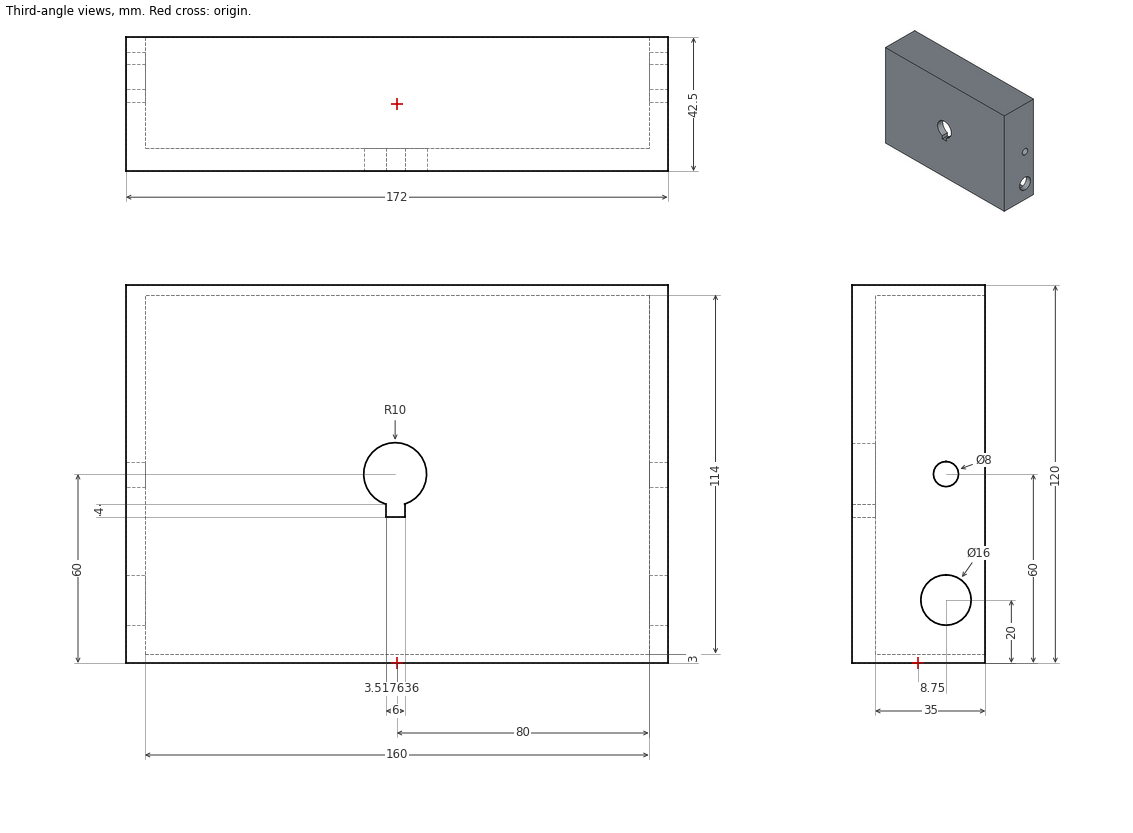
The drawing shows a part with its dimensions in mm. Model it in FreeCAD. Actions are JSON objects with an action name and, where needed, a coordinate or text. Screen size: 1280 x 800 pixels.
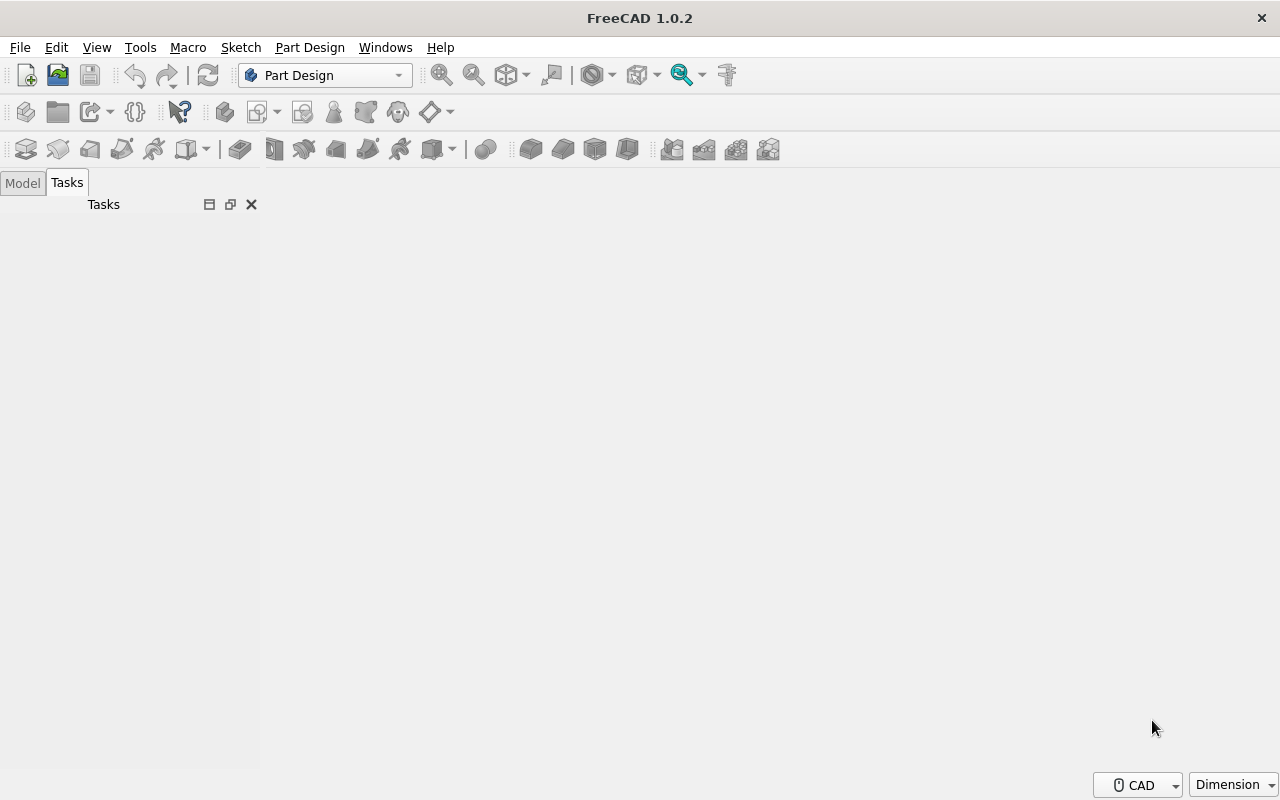
{"action": "left_click", "coordinate": [26, 76]}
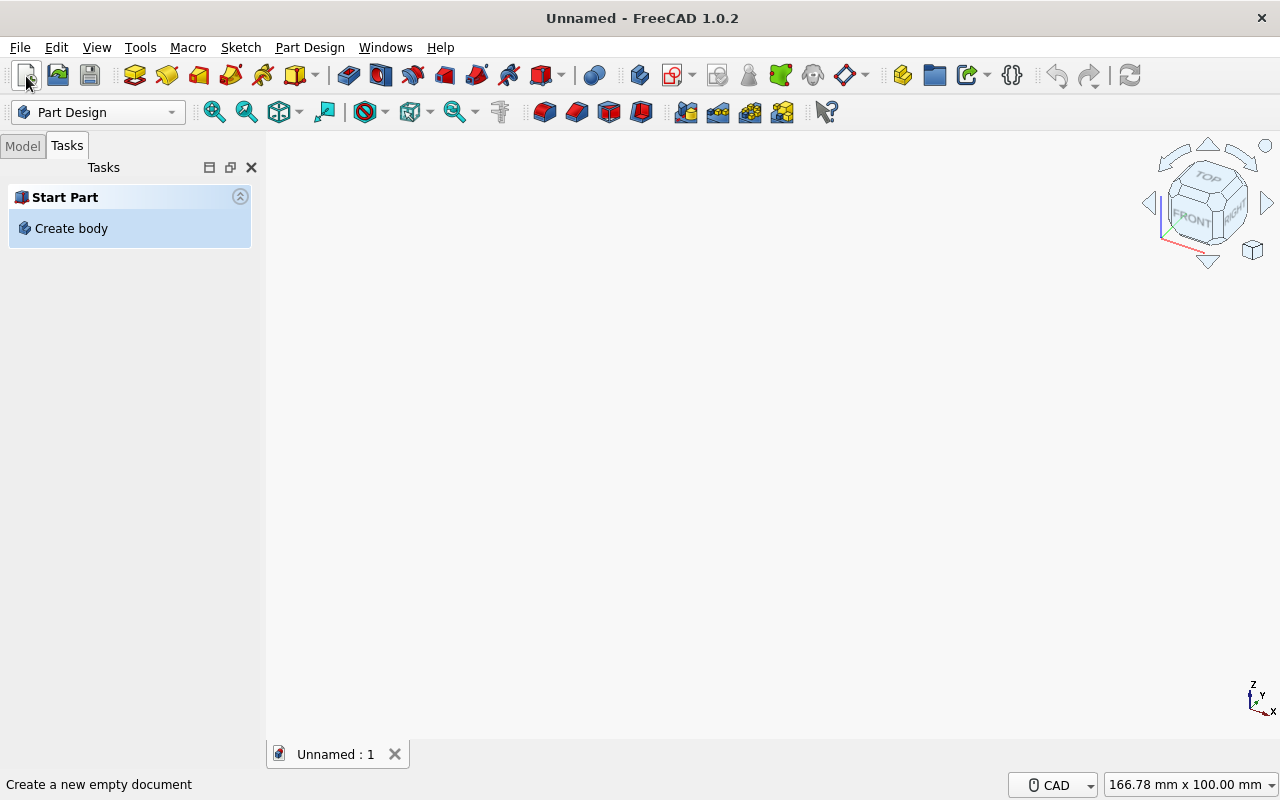
{"action": "left_click", "coordinate": [672, 76]}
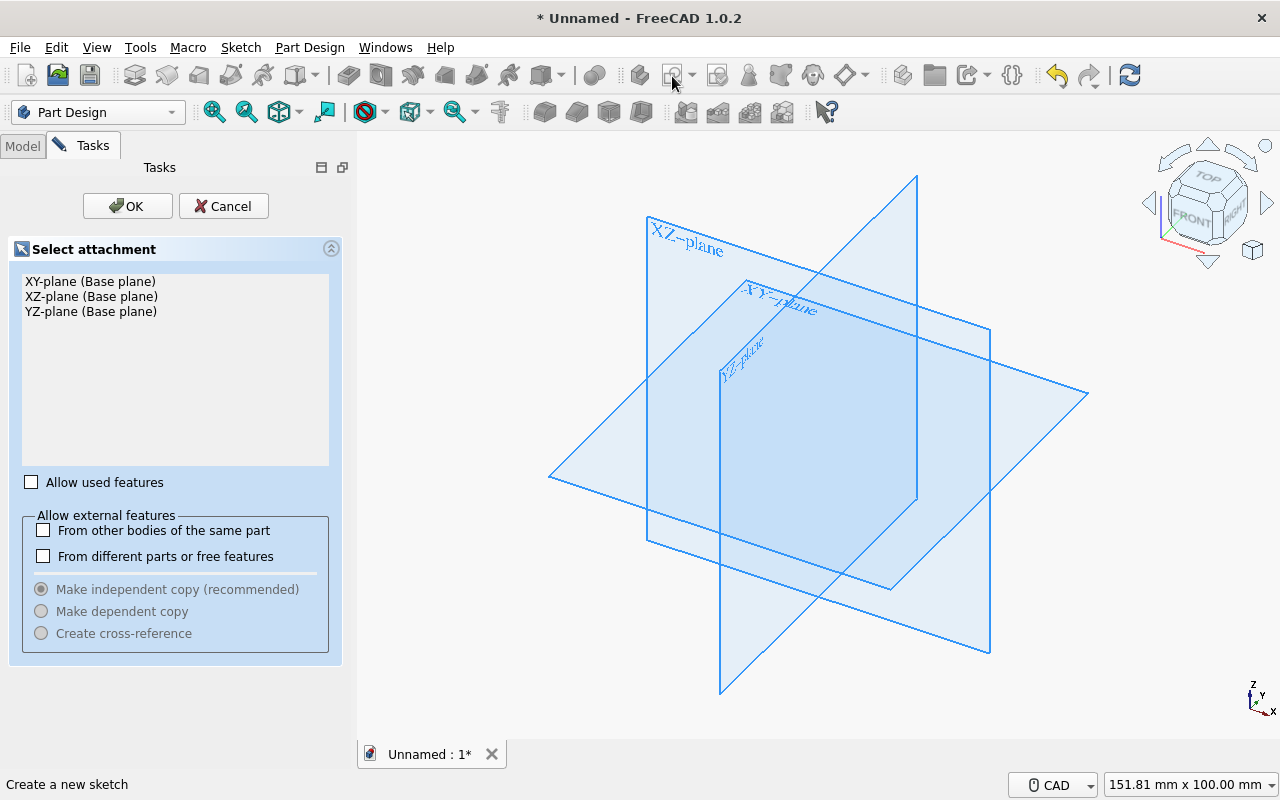
{"action": "left_click", "coordinate": [82, 282]}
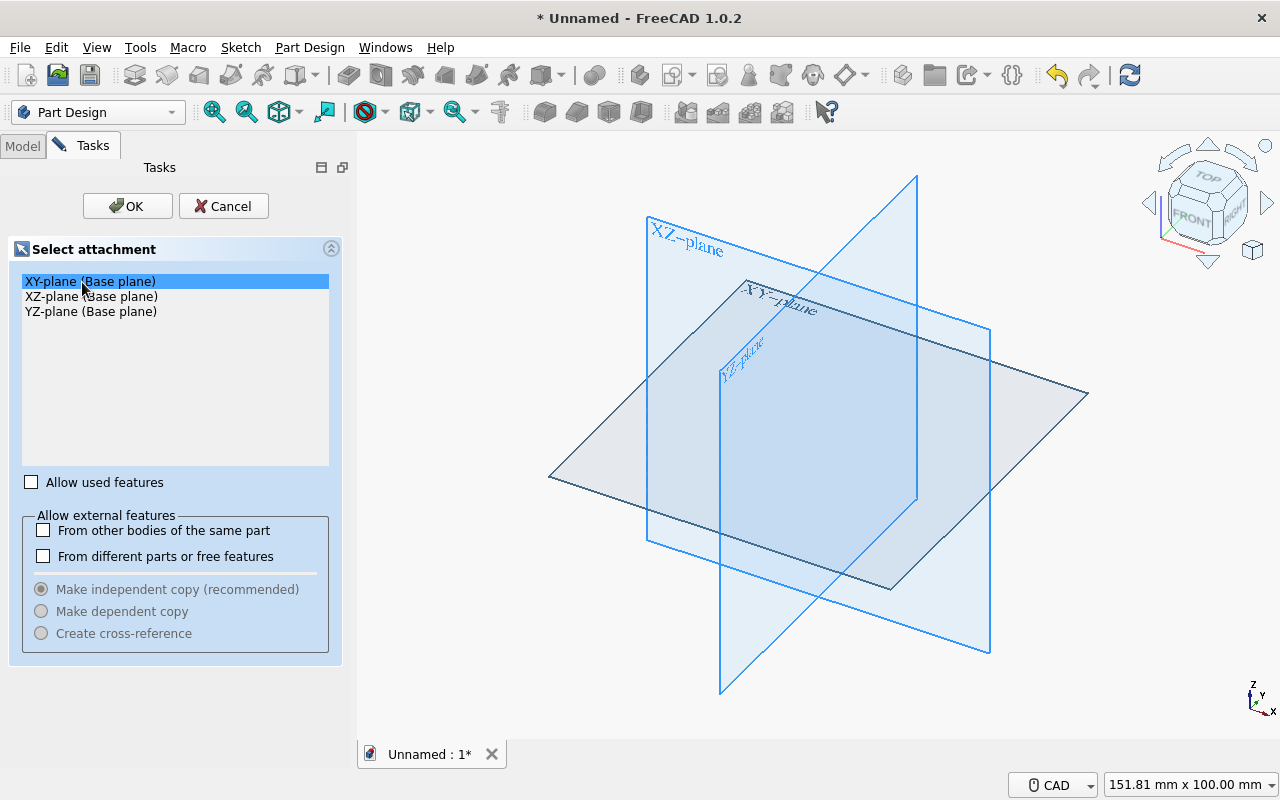
{"action": "left_click", "coordinate": [128, 206]}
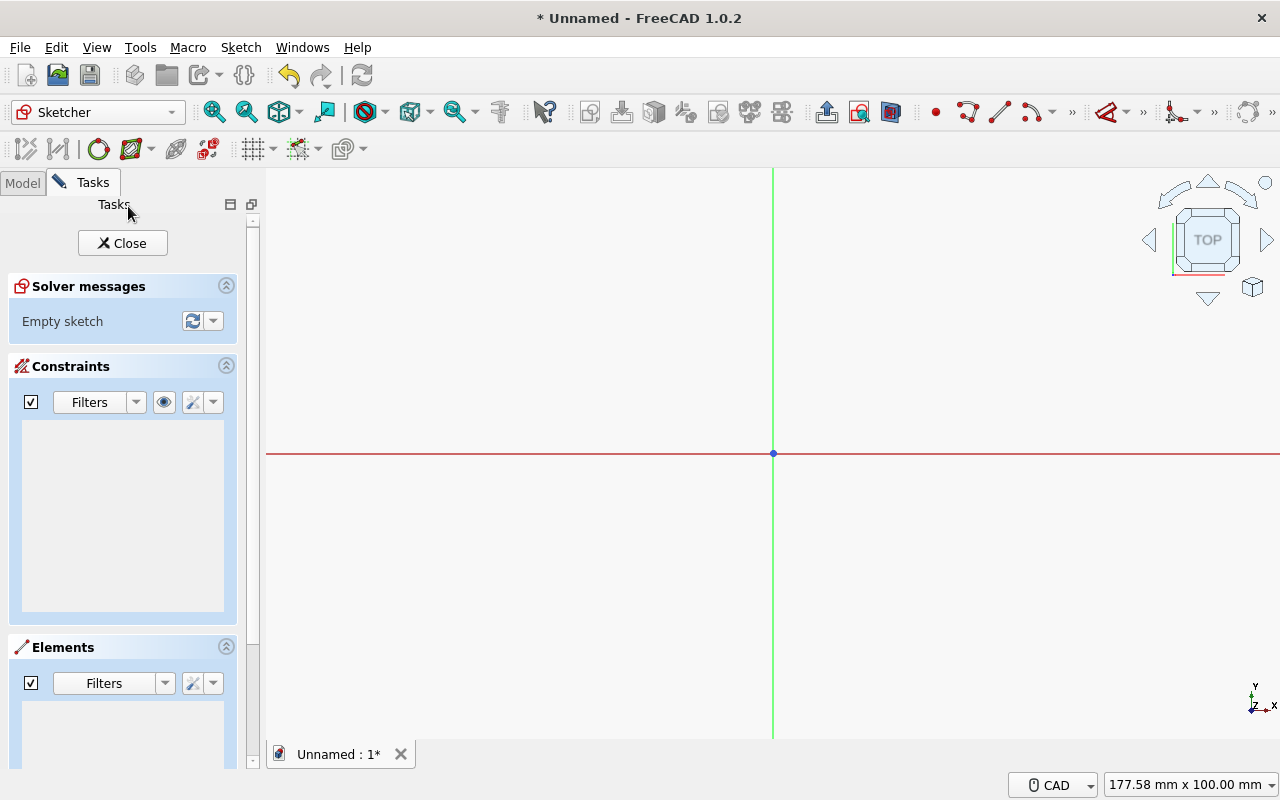
{"action": "scroll", "coordinate": [621, 454], "scroll_direction": "down", "scroll_amount": 3}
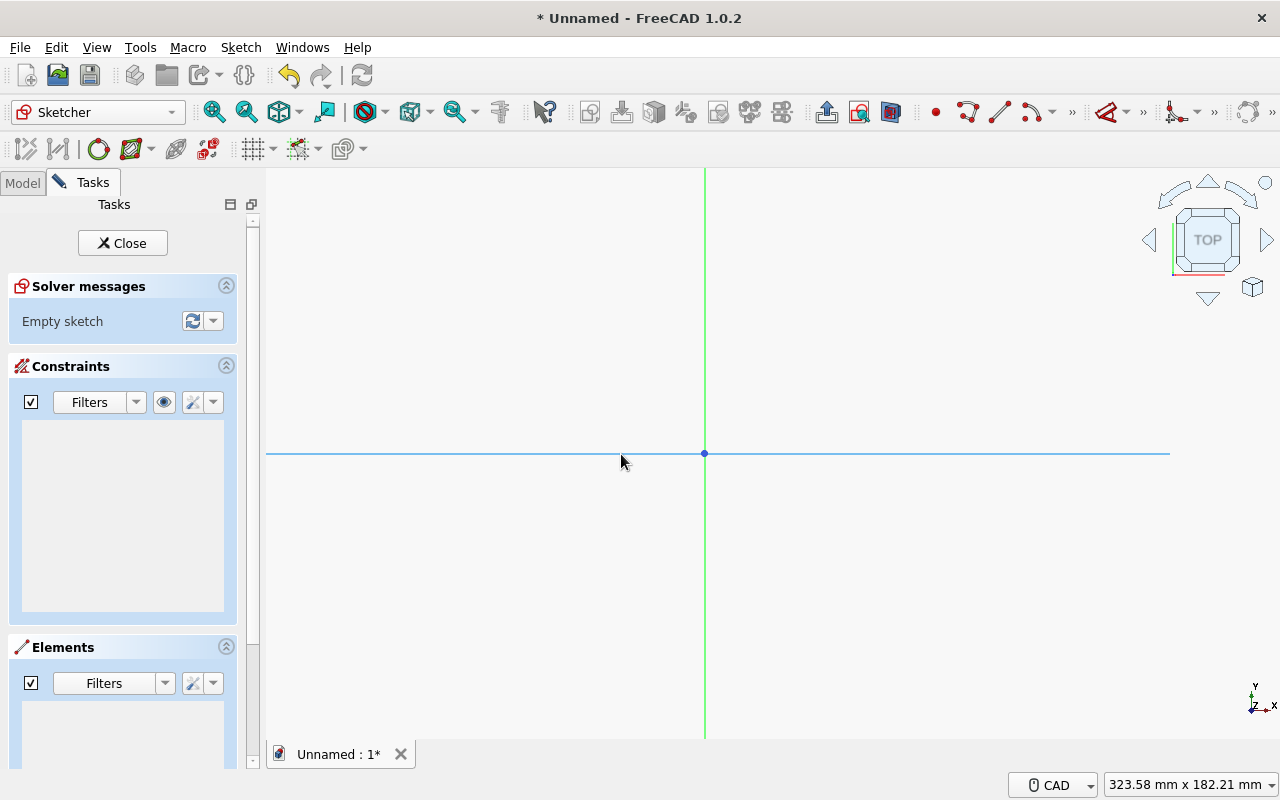
{"action": "key", "text": "g v"}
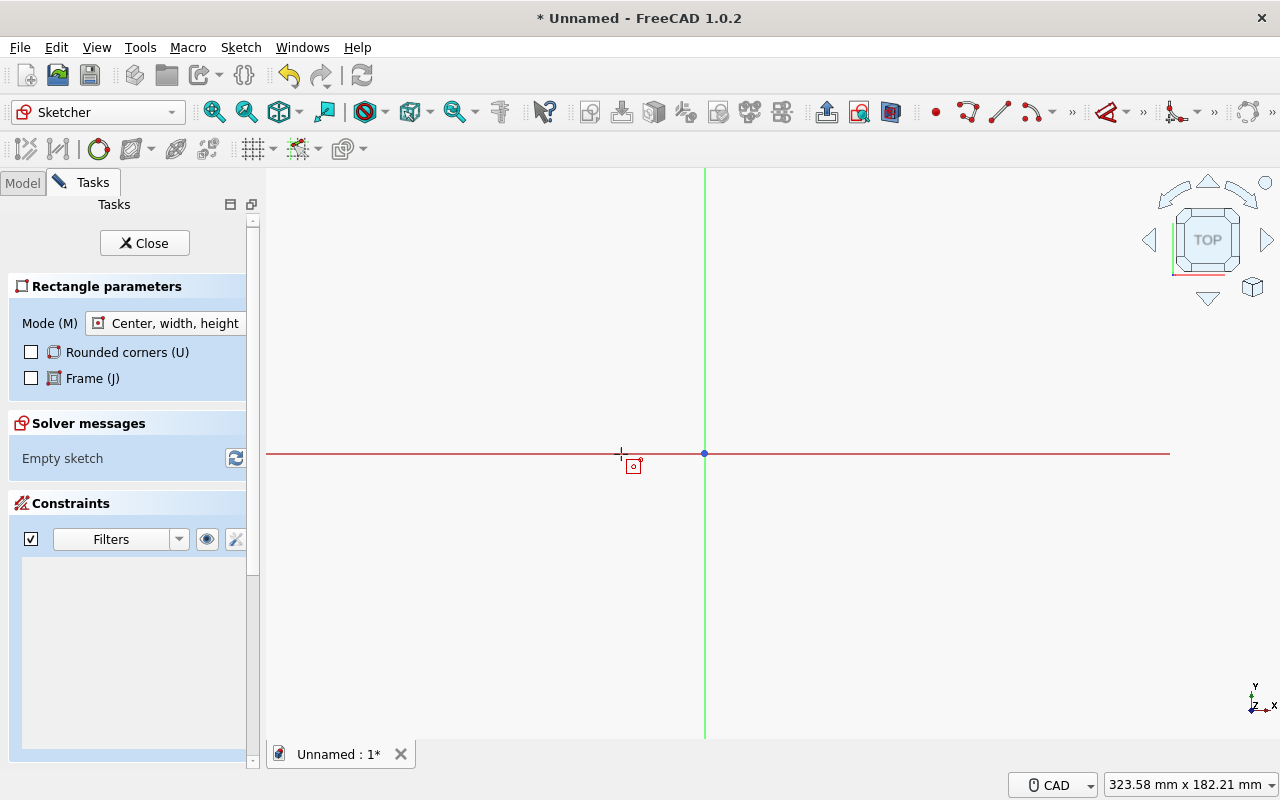
{"action": "left_click", "coordinate": [705, 454]}
{"action": "left_click", "coordinate": [974, 387]}
{"action": "key", "text": "Escape"}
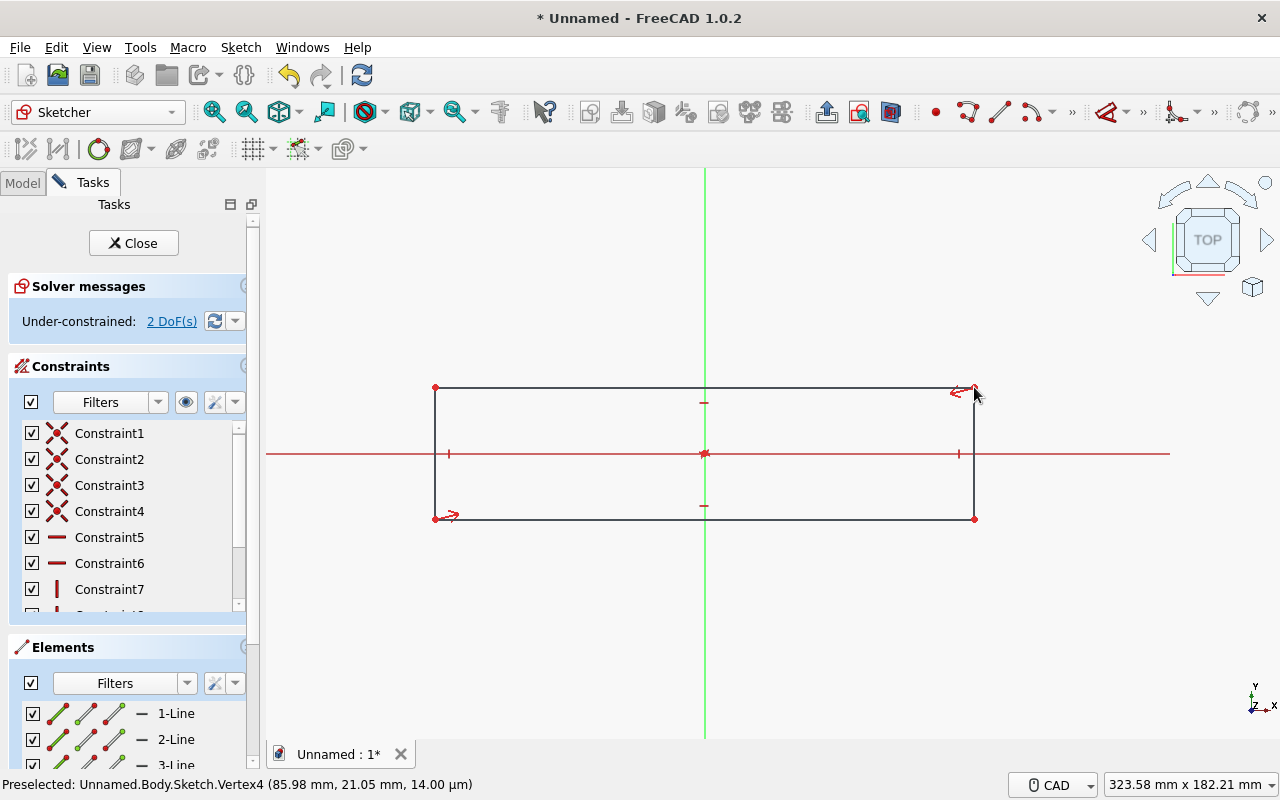
{"action": "left_click", "coordinate": [1106, 112]}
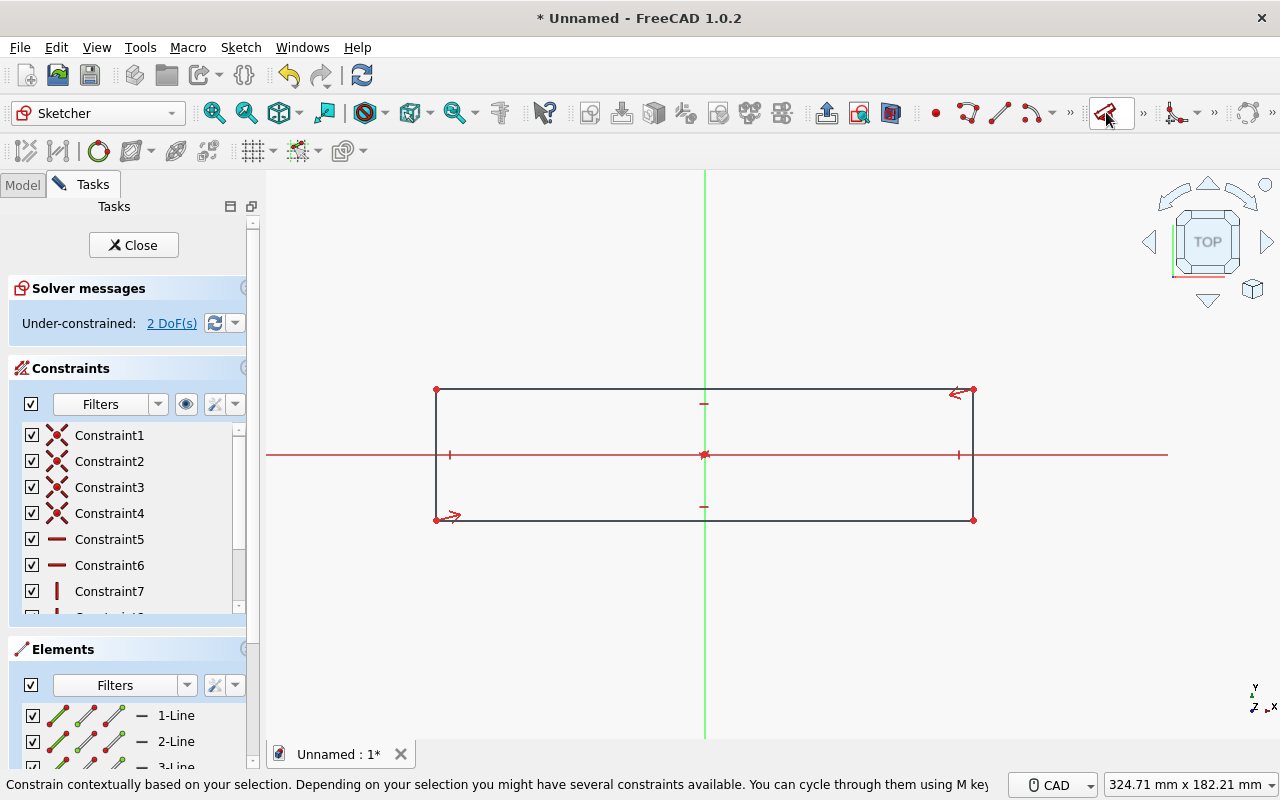
{"action": "left_click", "coordinate": [597, 521]}
{"action": "left_click", "coordinate": [581, 555]}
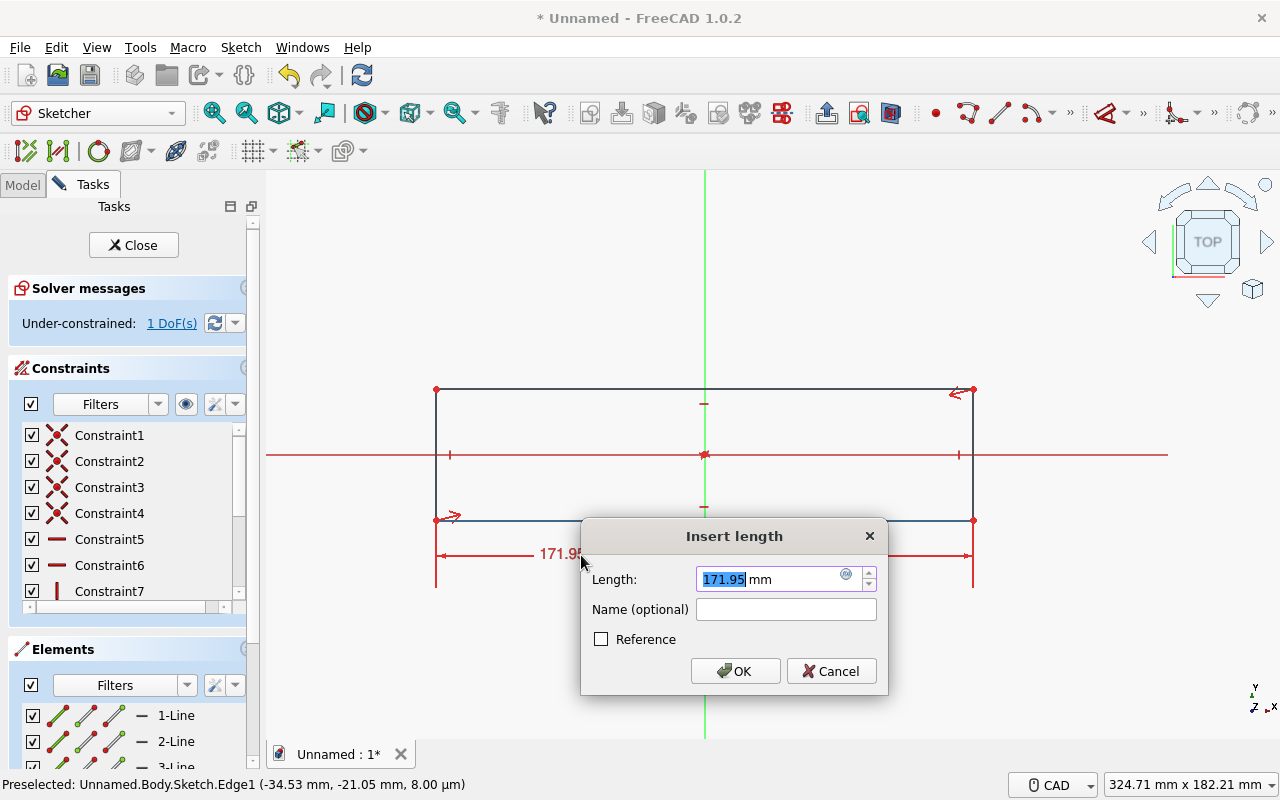
{"action": "type", "text": "172"}
{"action": "key", "text": "Return"}